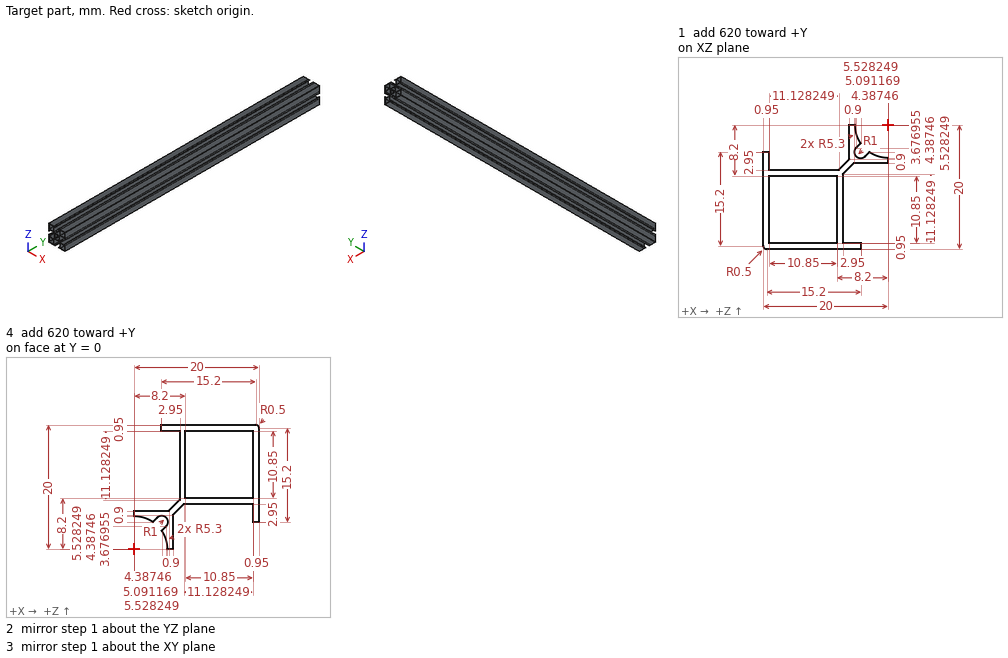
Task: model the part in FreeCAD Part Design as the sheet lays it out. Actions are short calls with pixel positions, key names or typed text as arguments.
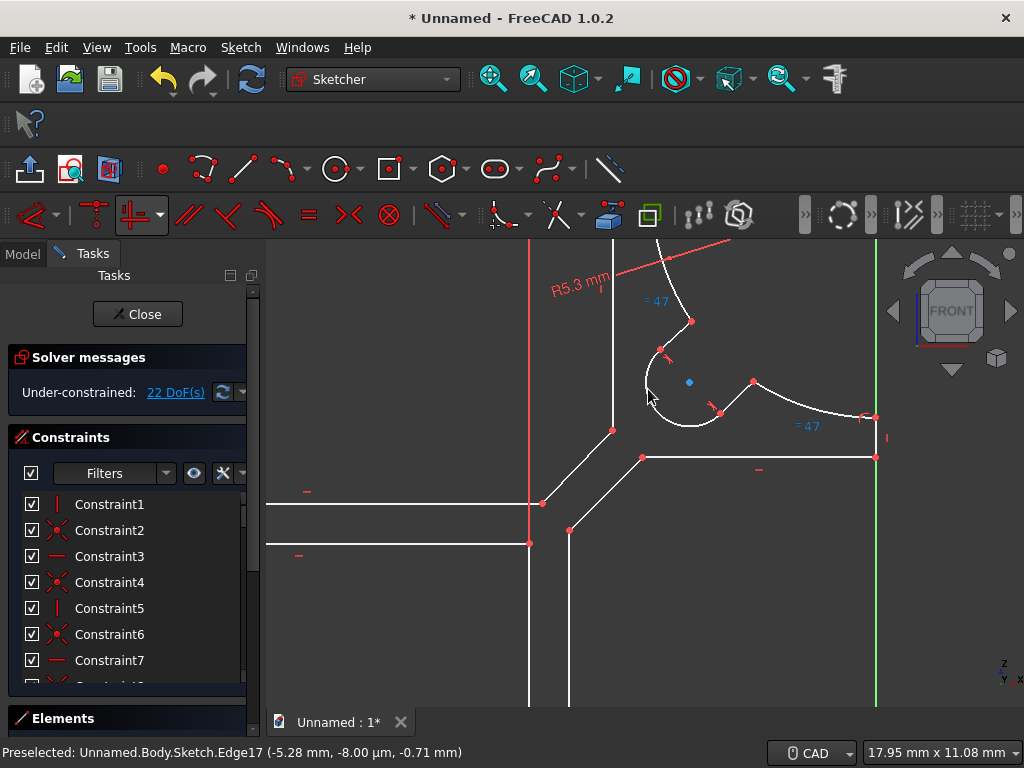
click(646, 388)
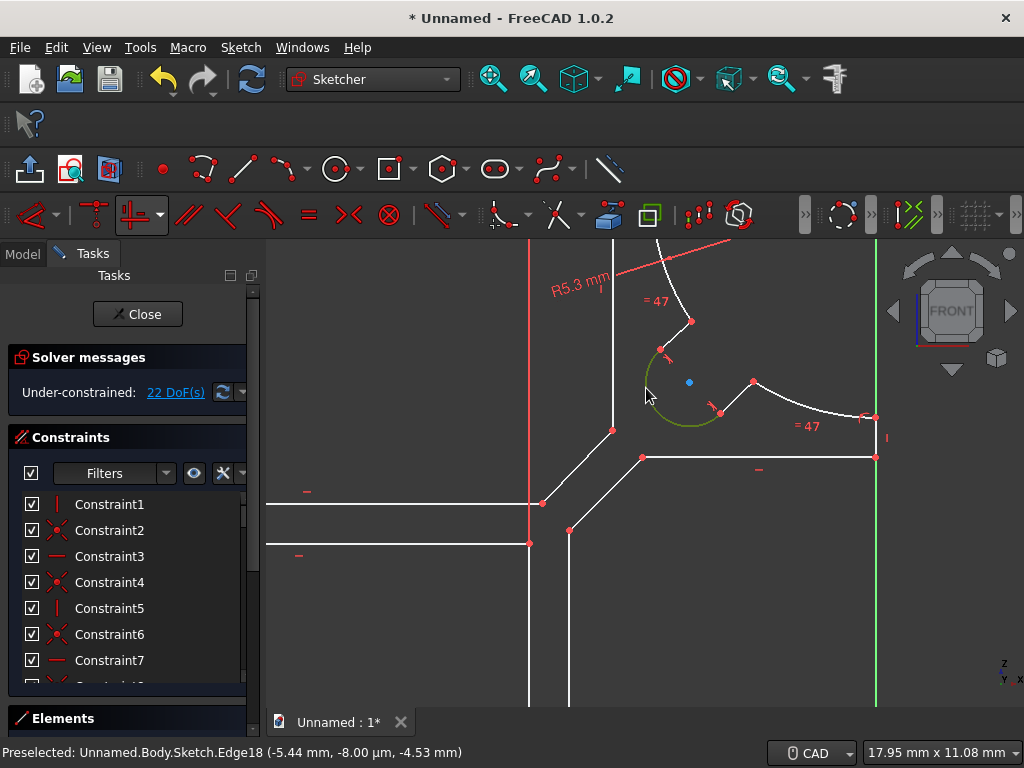
key(k)
key(r)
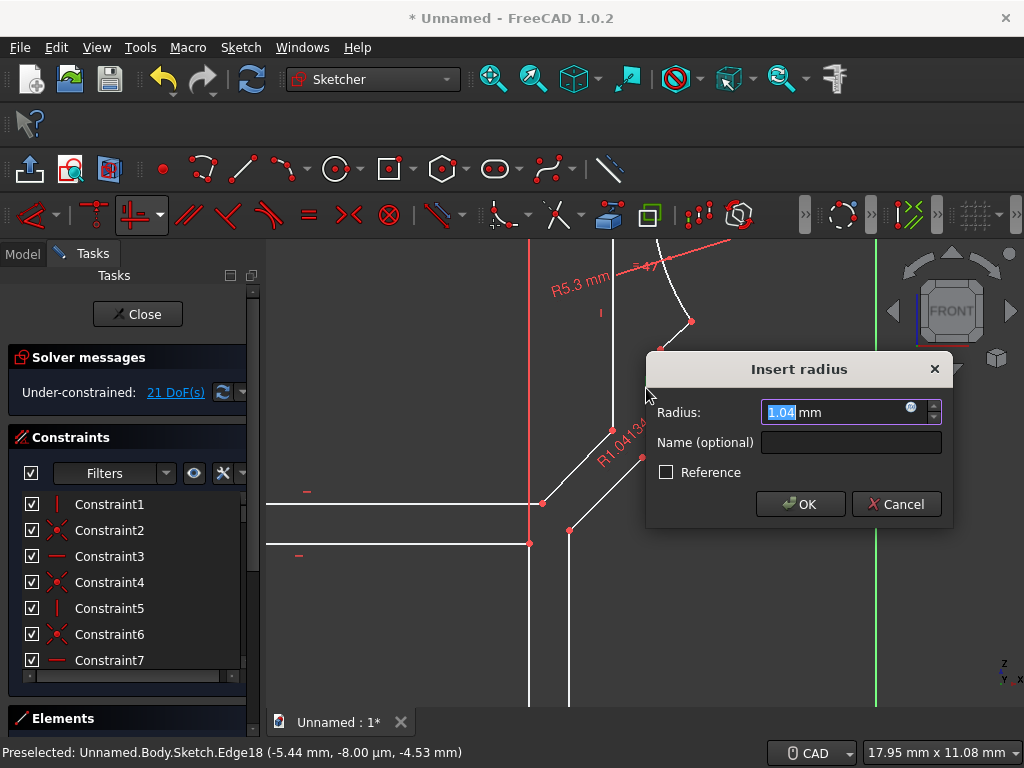
text(1)
key(Return)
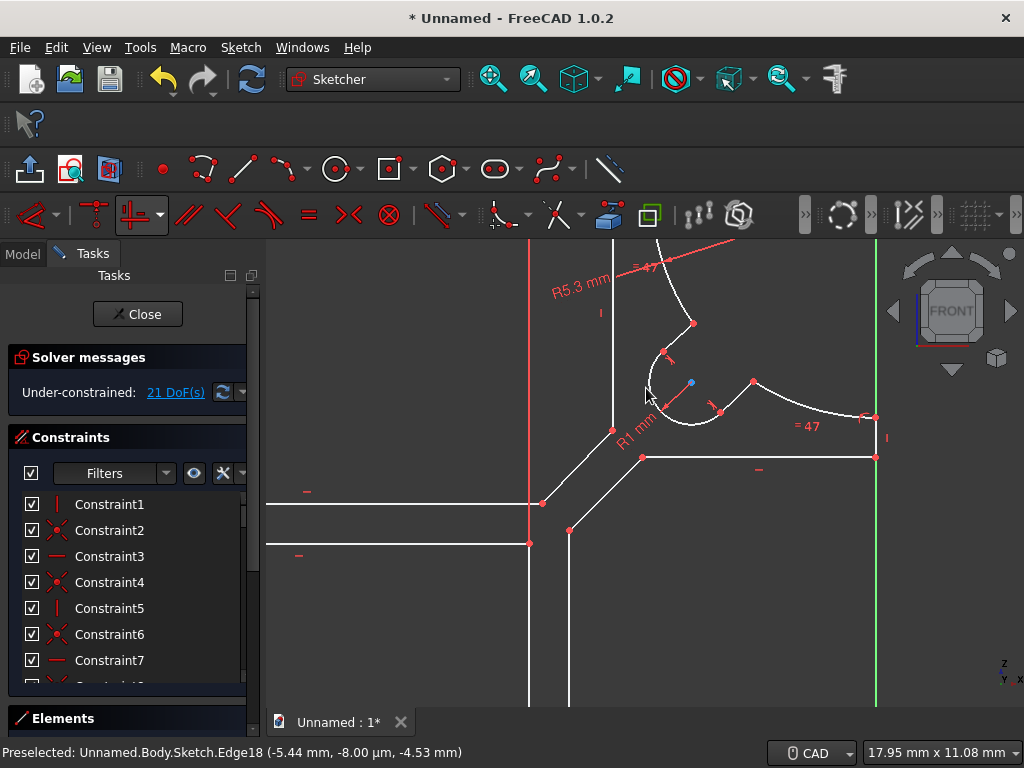
scroll(648, 390, down, 5)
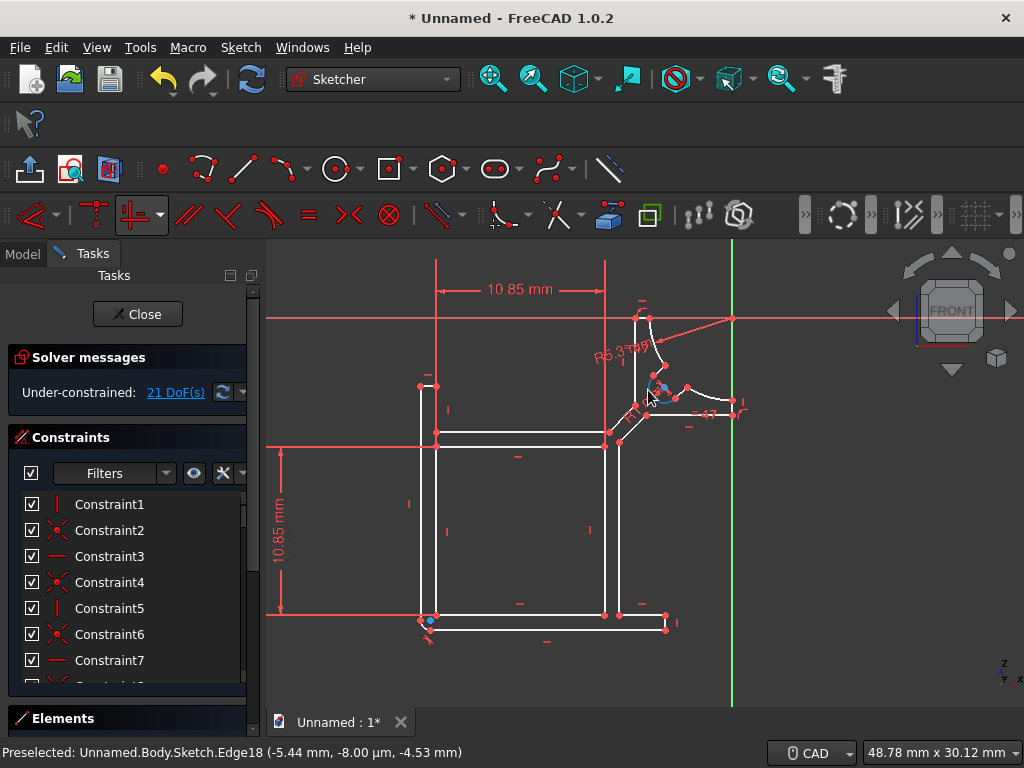
scroll(422, 625, up, 9)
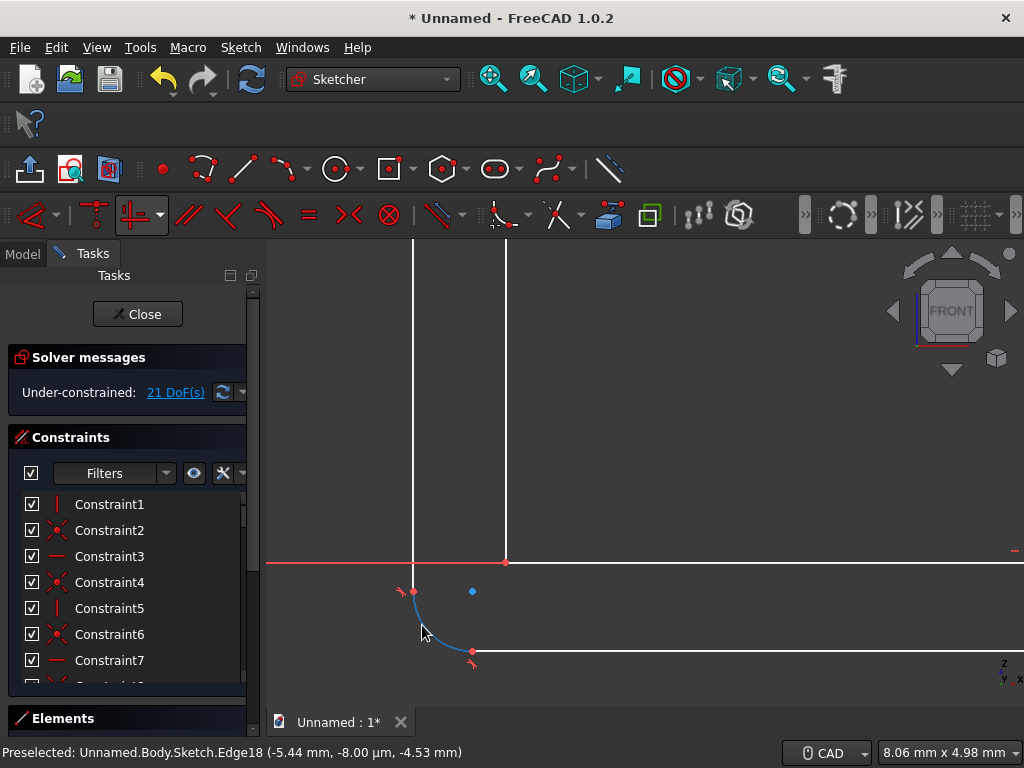
click(420, 619)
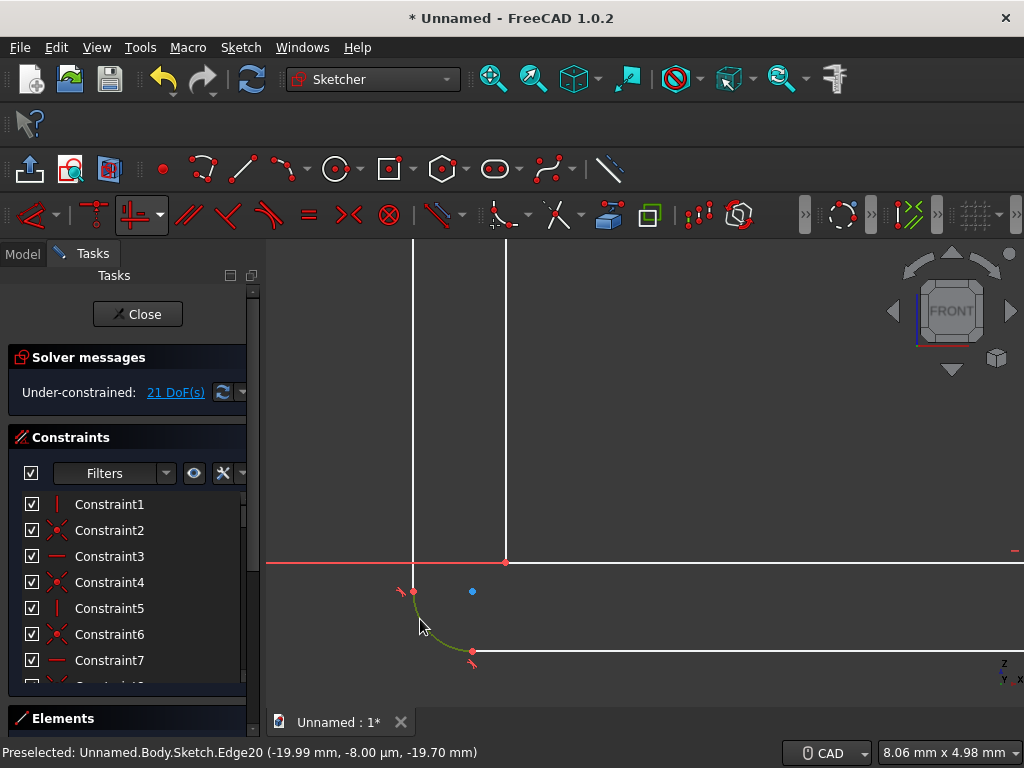
key(k)
key(r)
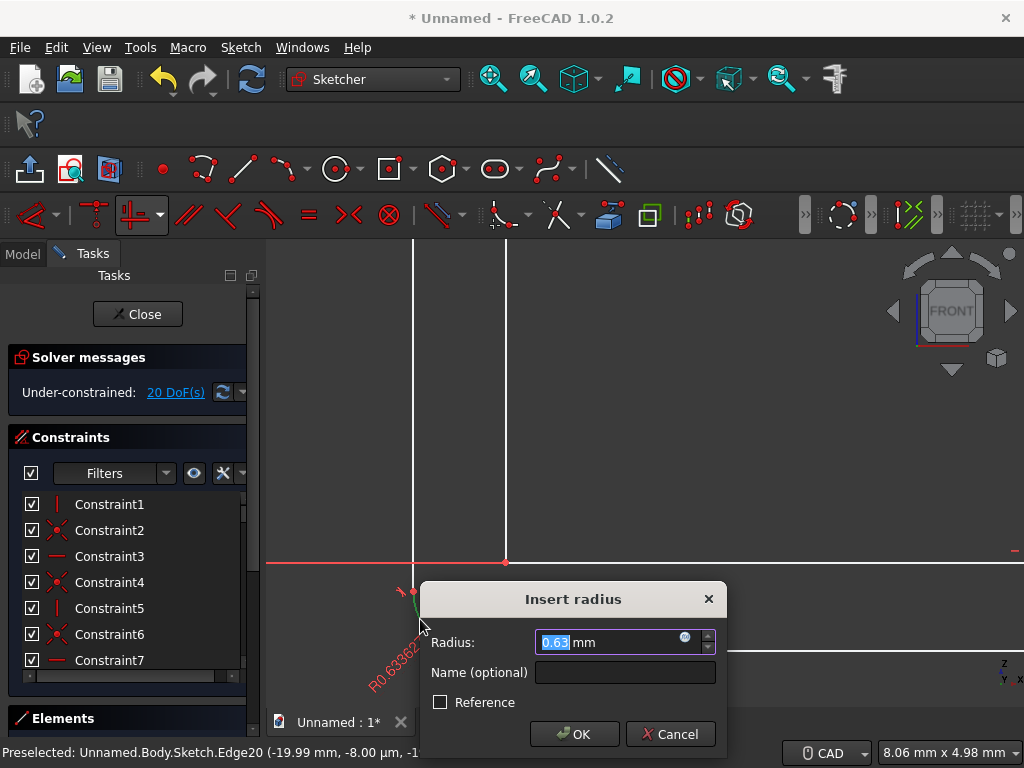
text(0.5)
key(Return)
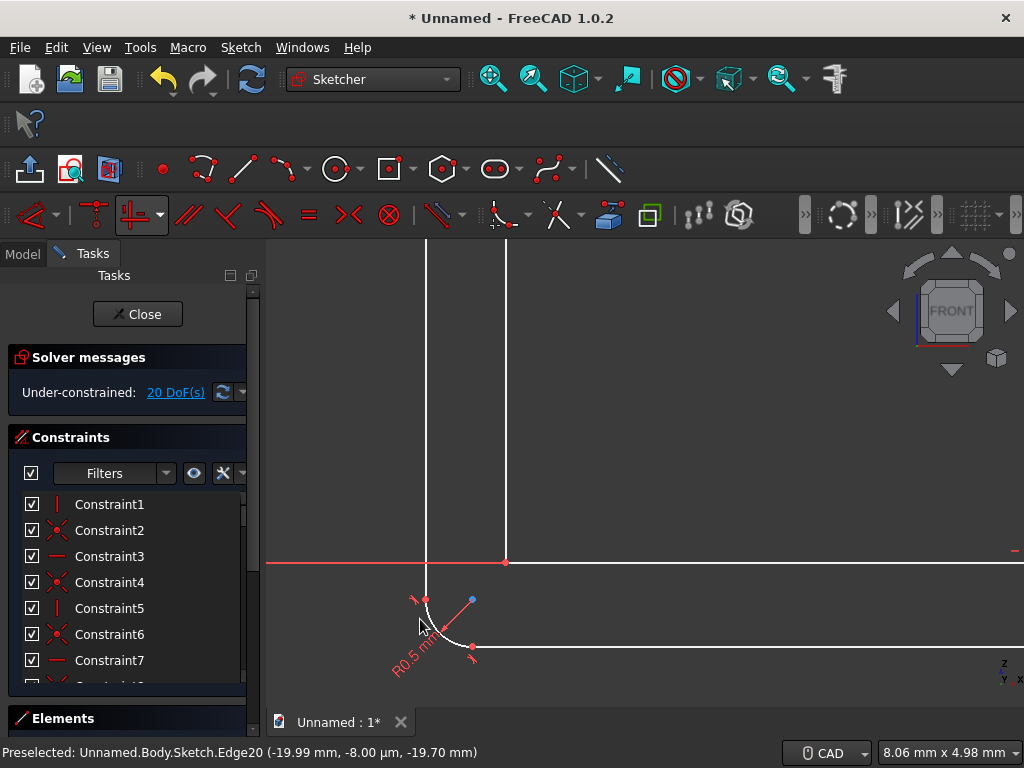
scroll(422, 625, down, 9)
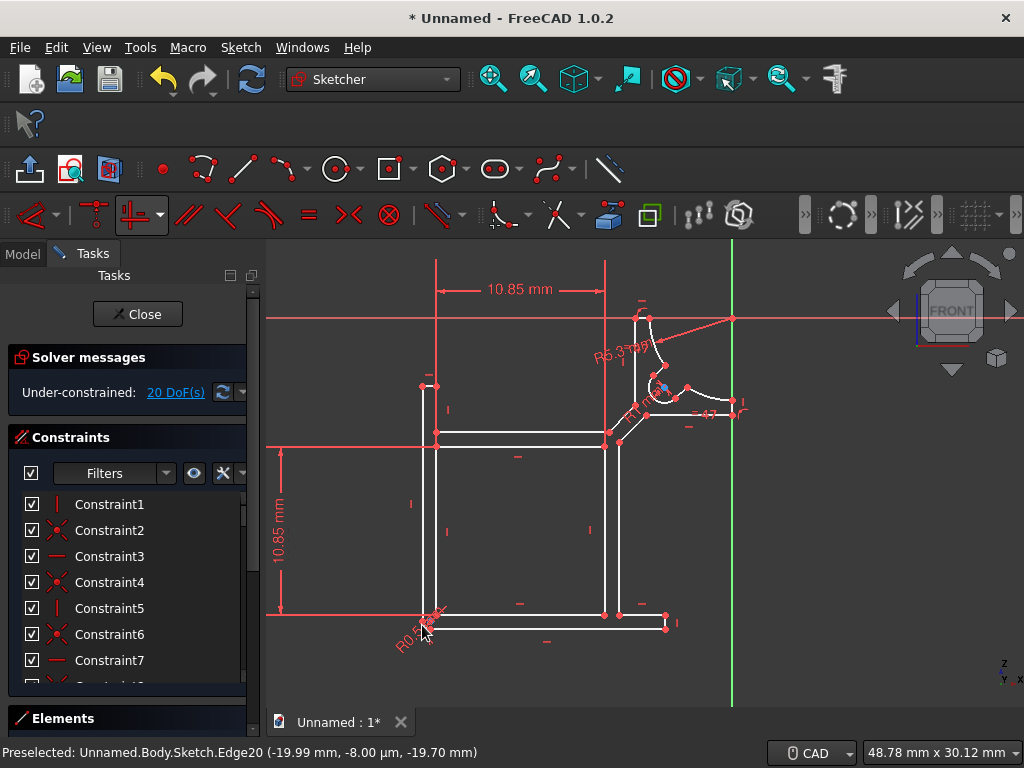
scroll(640, 318, up, 6)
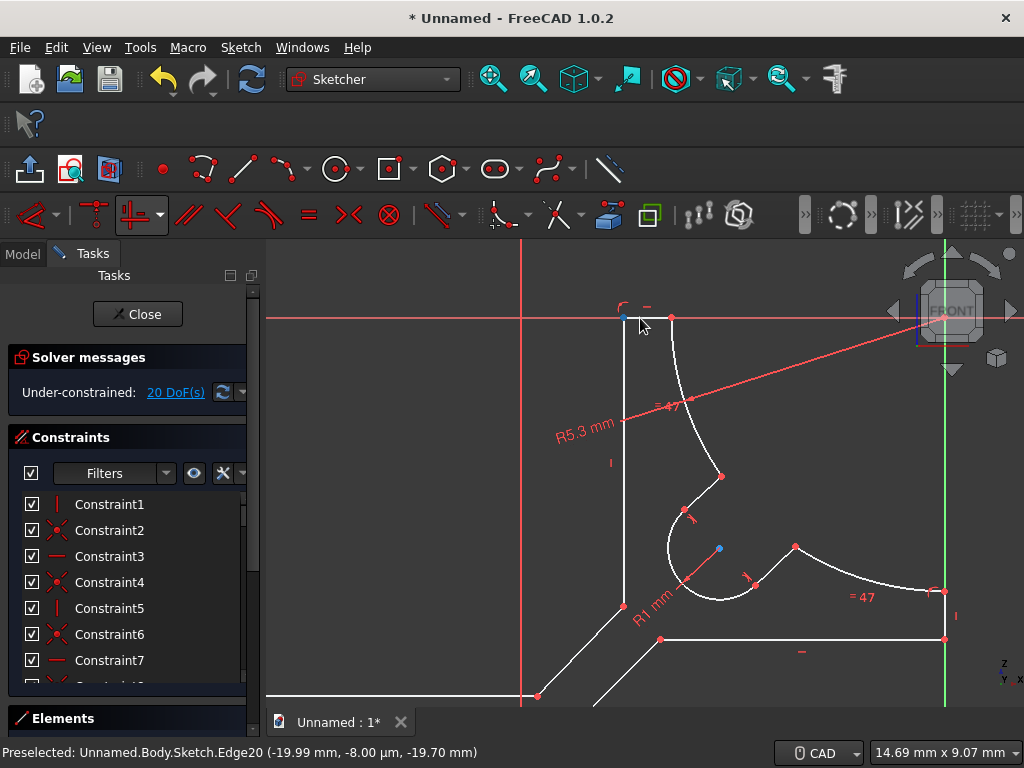
click(638, 318)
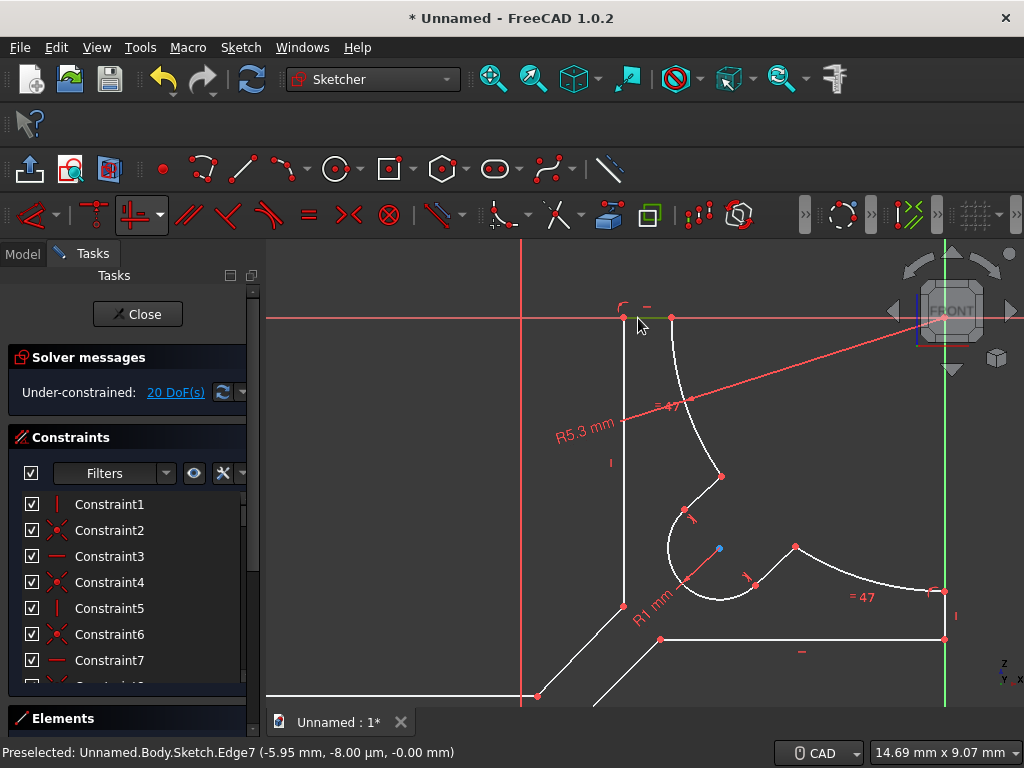
click(58, 216)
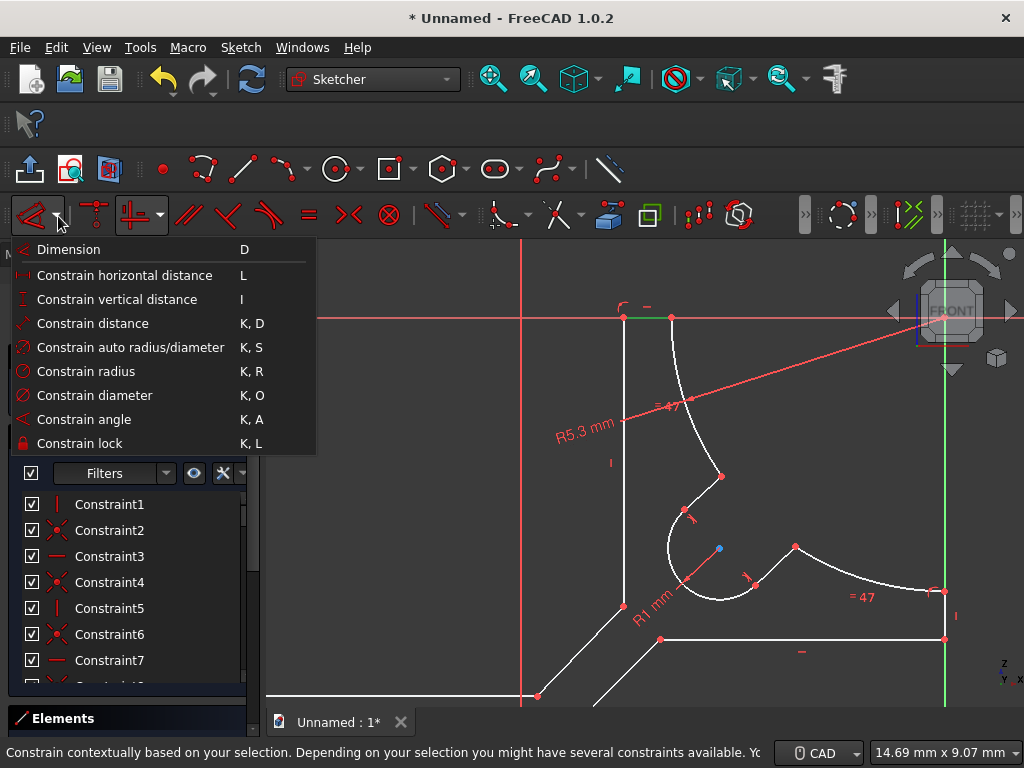
click(164, 275)